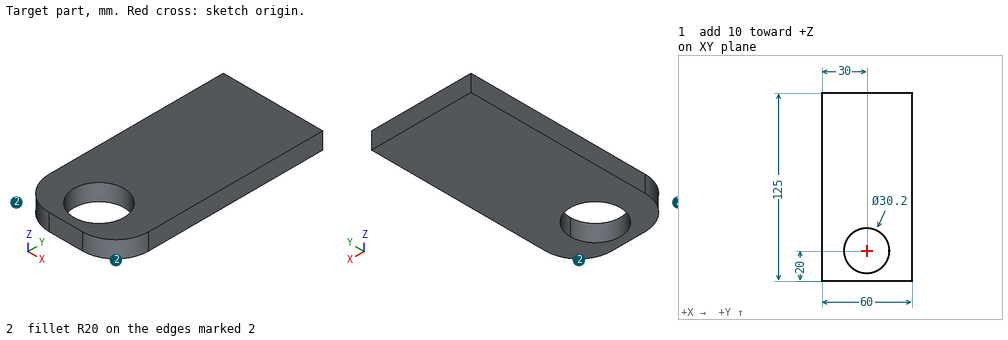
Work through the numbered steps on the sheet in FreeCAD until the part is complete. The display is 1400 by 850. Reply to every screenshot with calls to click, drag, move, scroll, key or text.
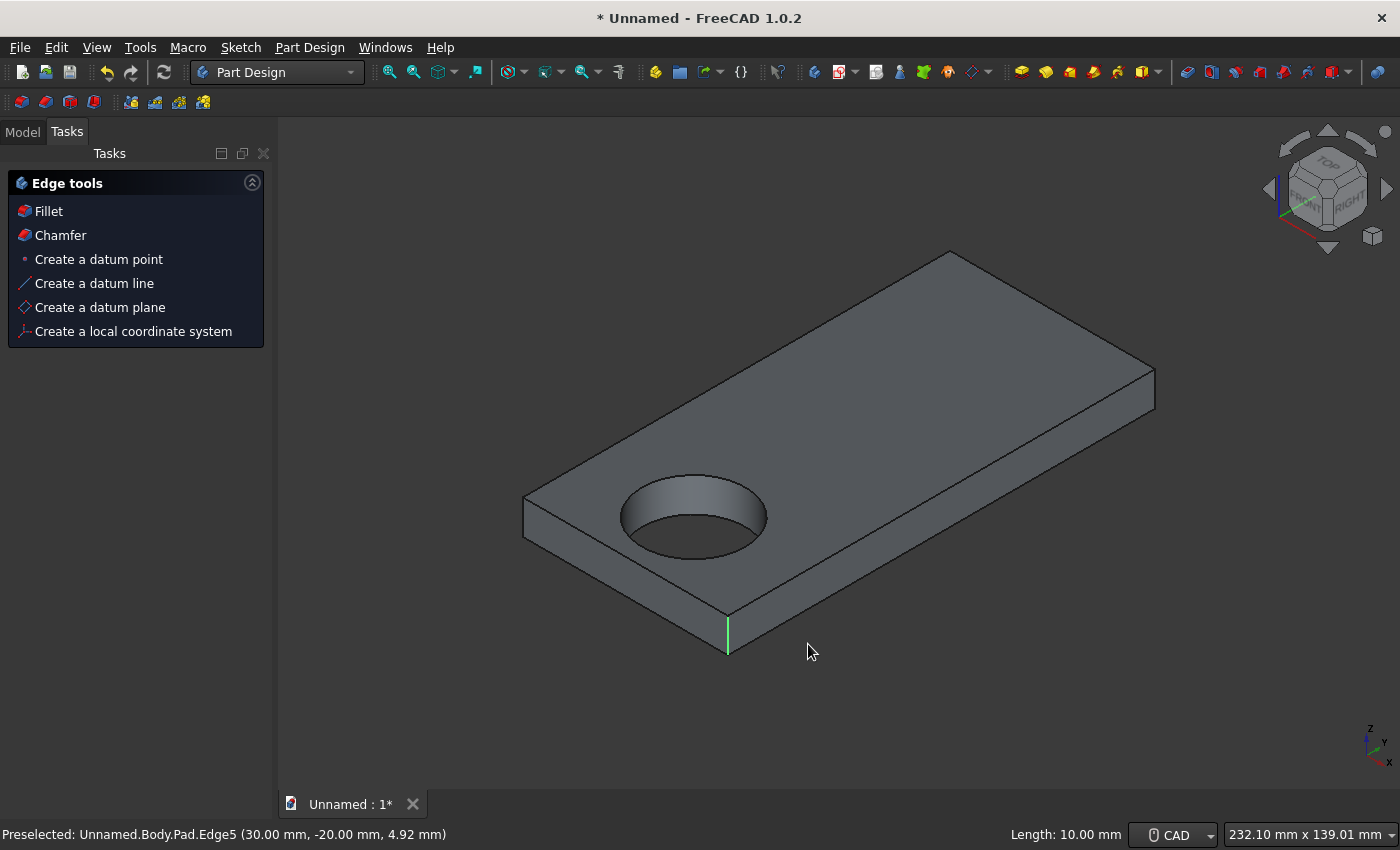
key(2)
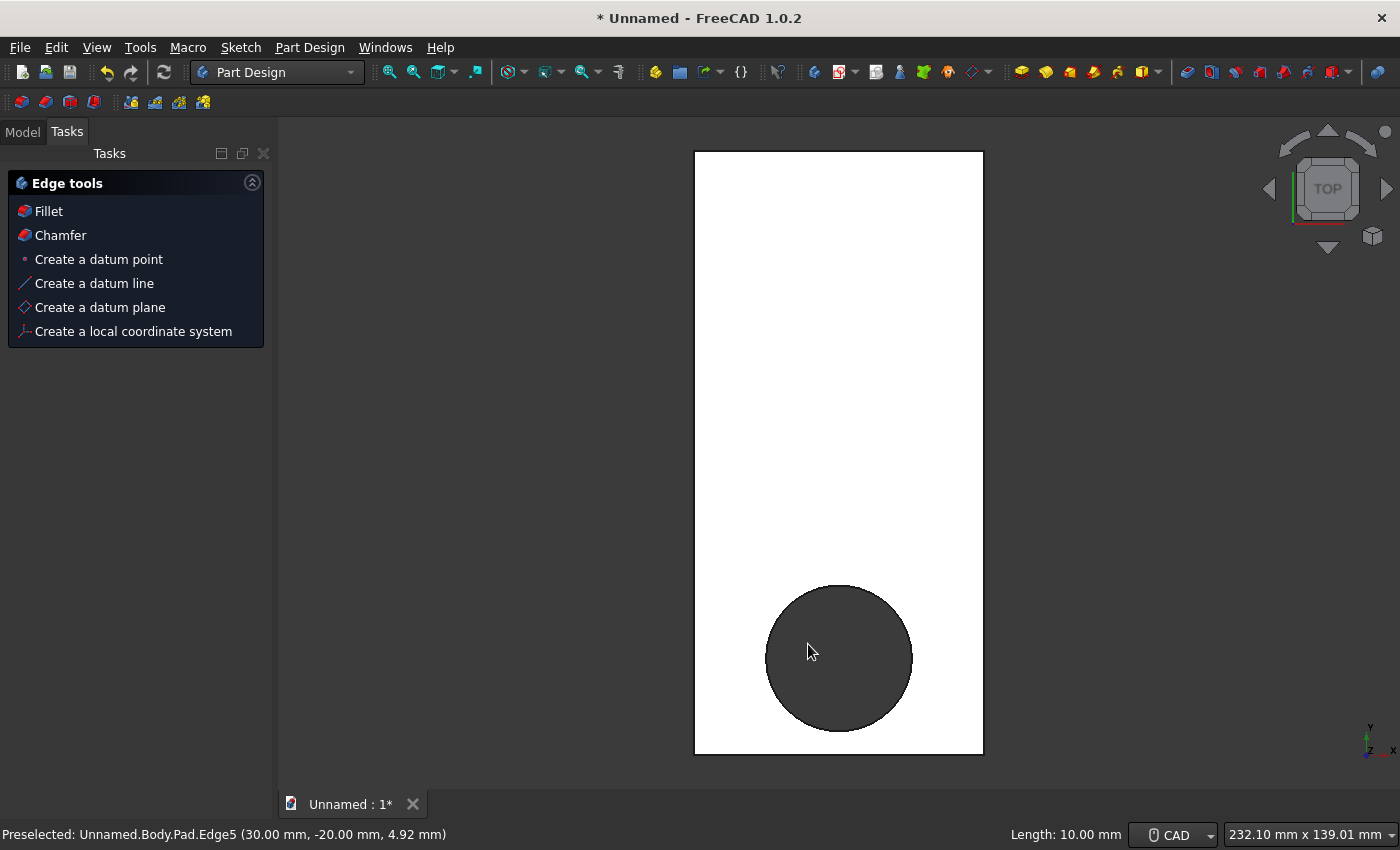
key(1)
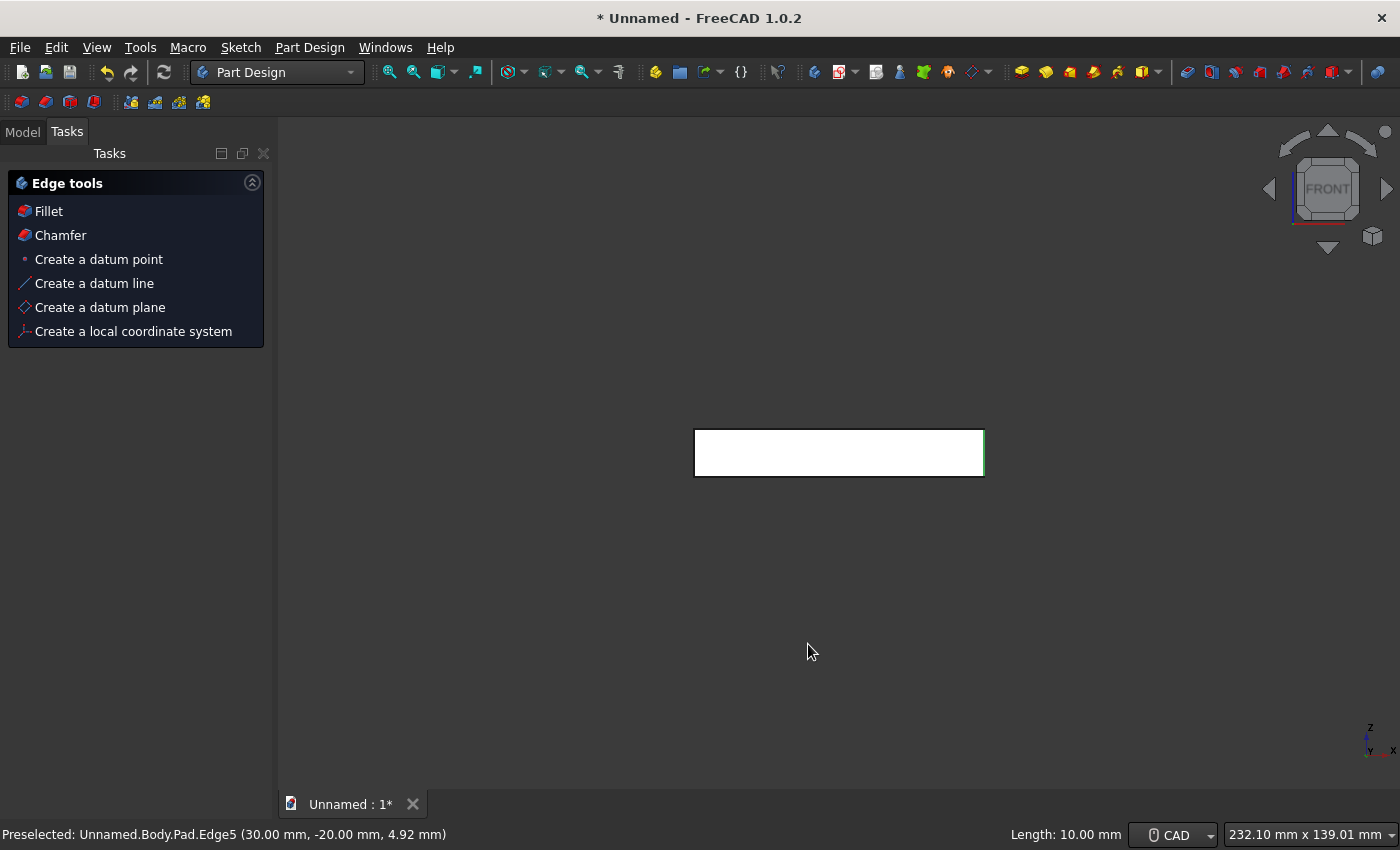
click(390, 72)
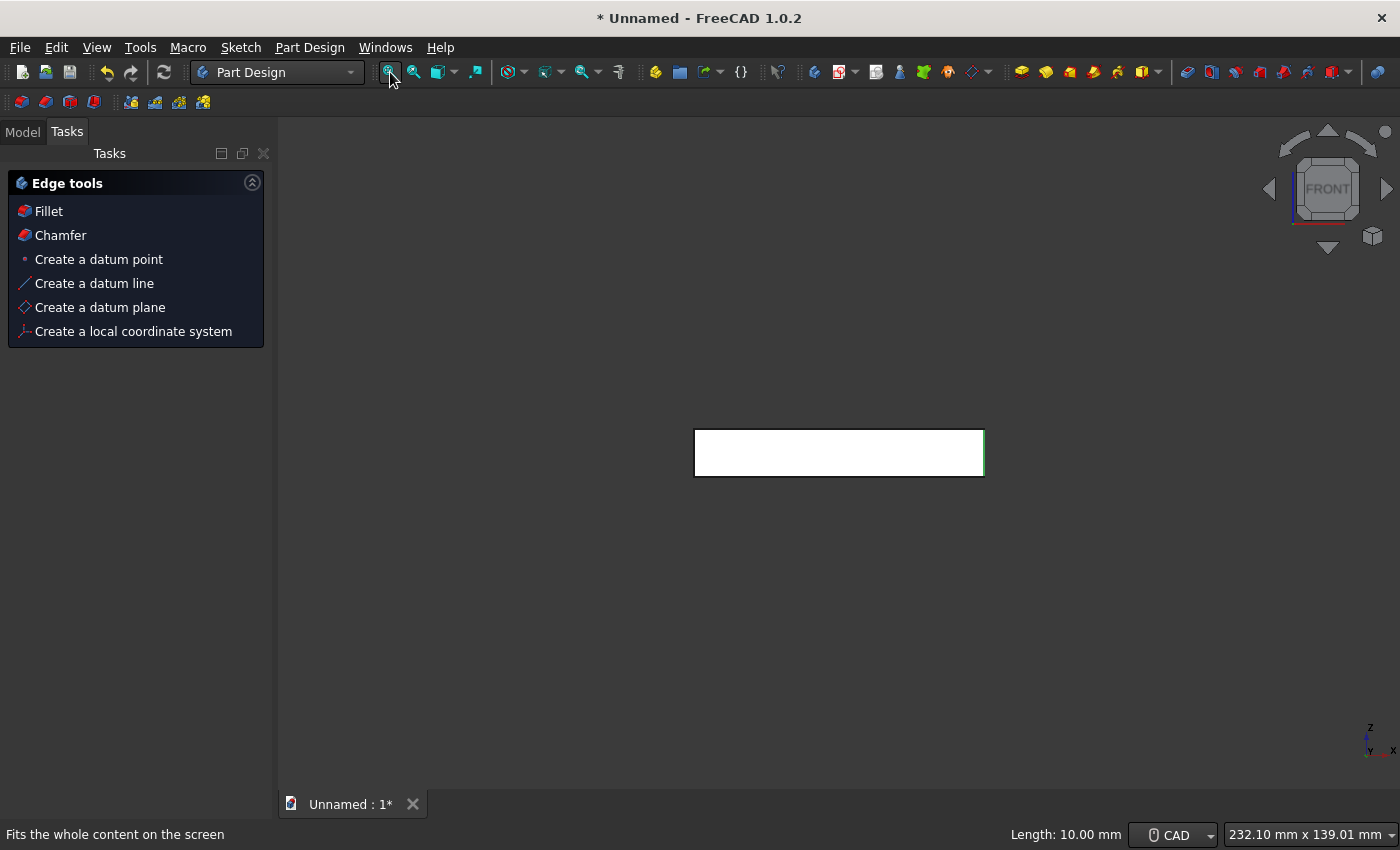
click(694, 452, ctrl)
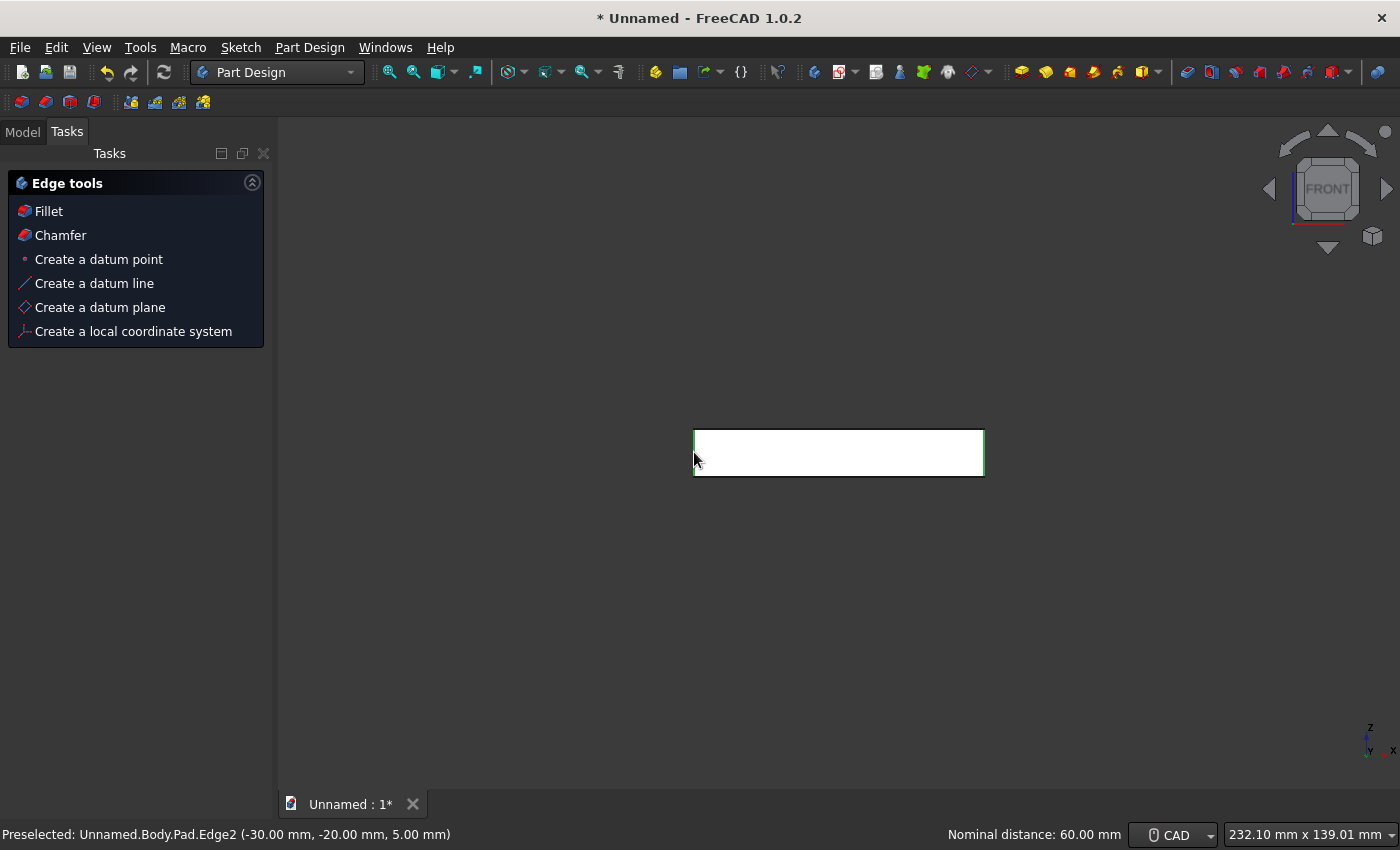
click(22, 102)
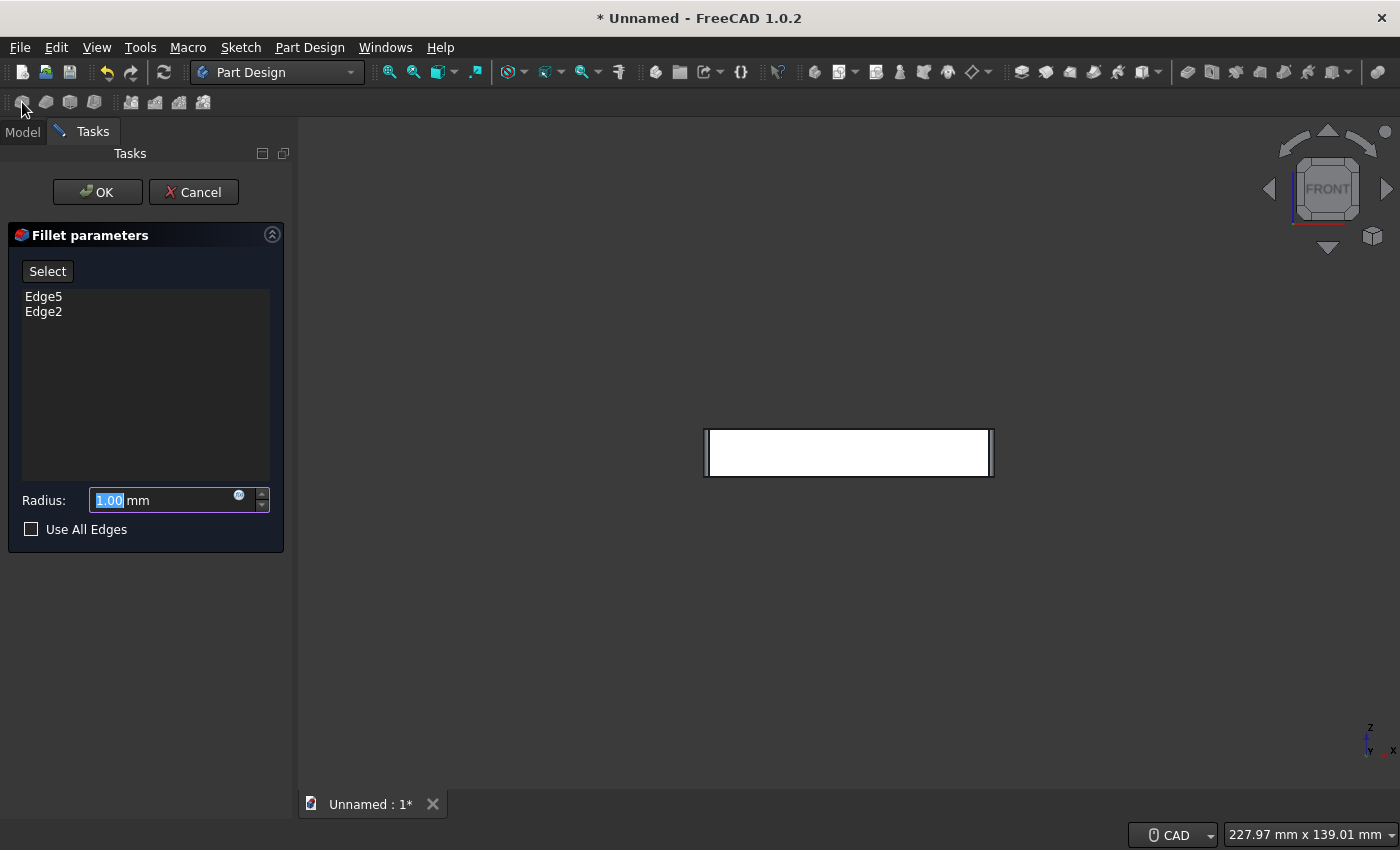
text(20)
key(Tab)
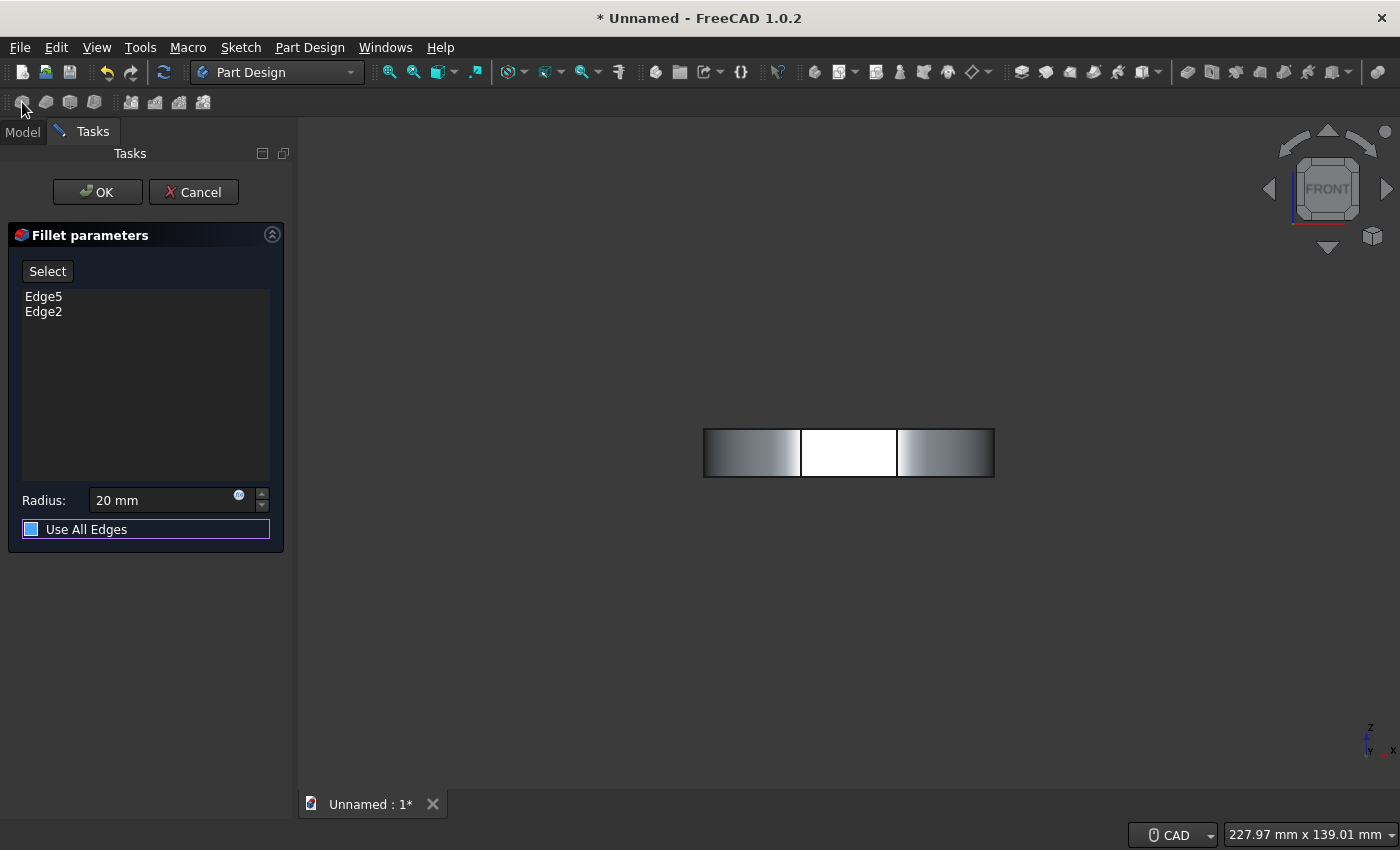
click(98, 192)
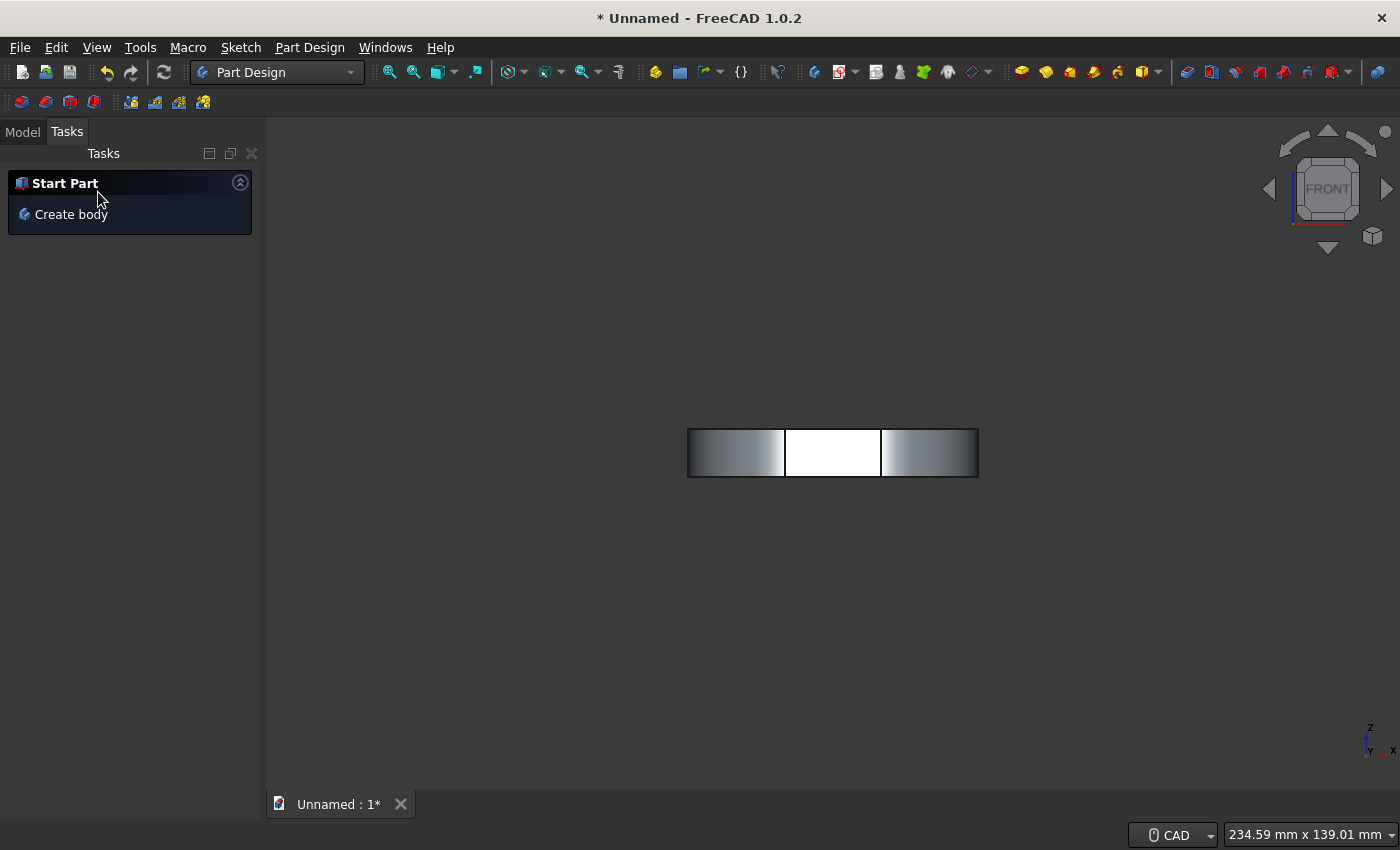
key(0)